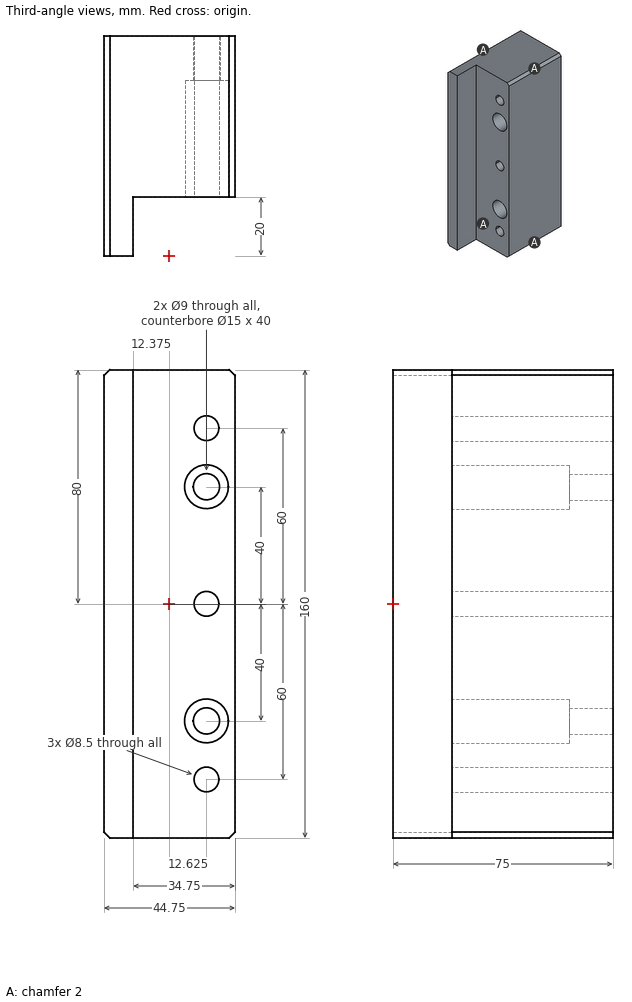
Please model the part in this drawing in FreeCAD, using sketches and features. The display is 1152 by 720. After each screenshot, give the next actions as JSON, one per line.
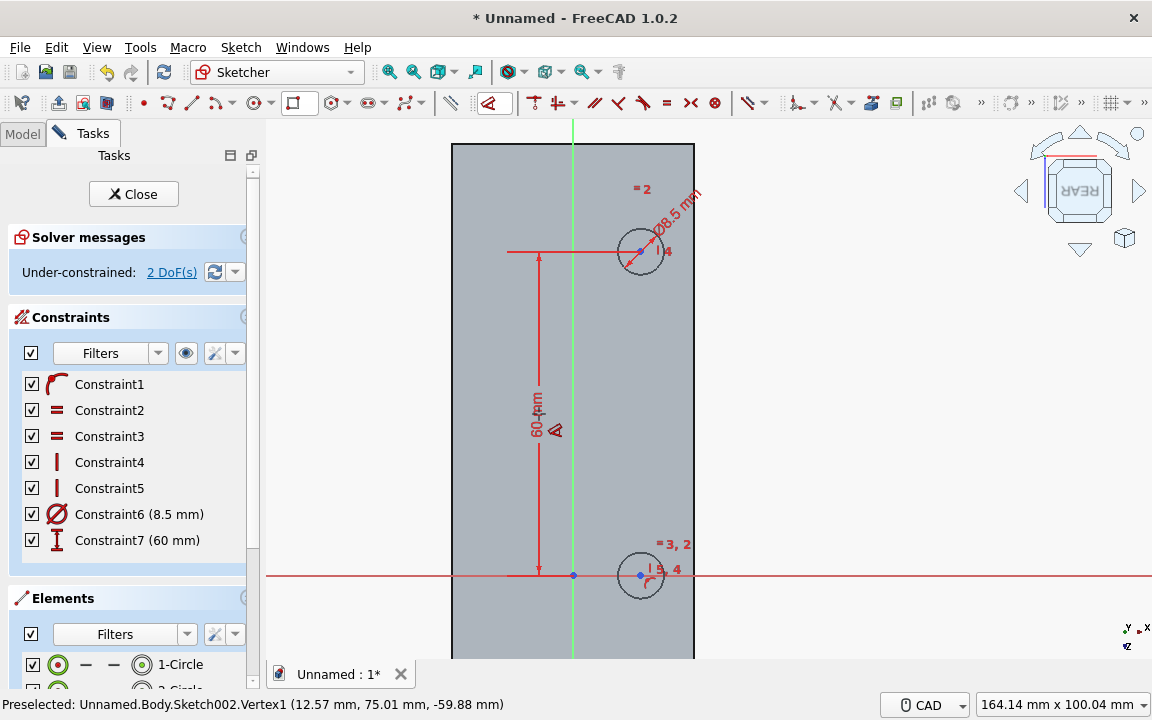
{"action": "scroll", "coordinate": [658, 237], "scroll_direction": "down", "scroll_amount": 4}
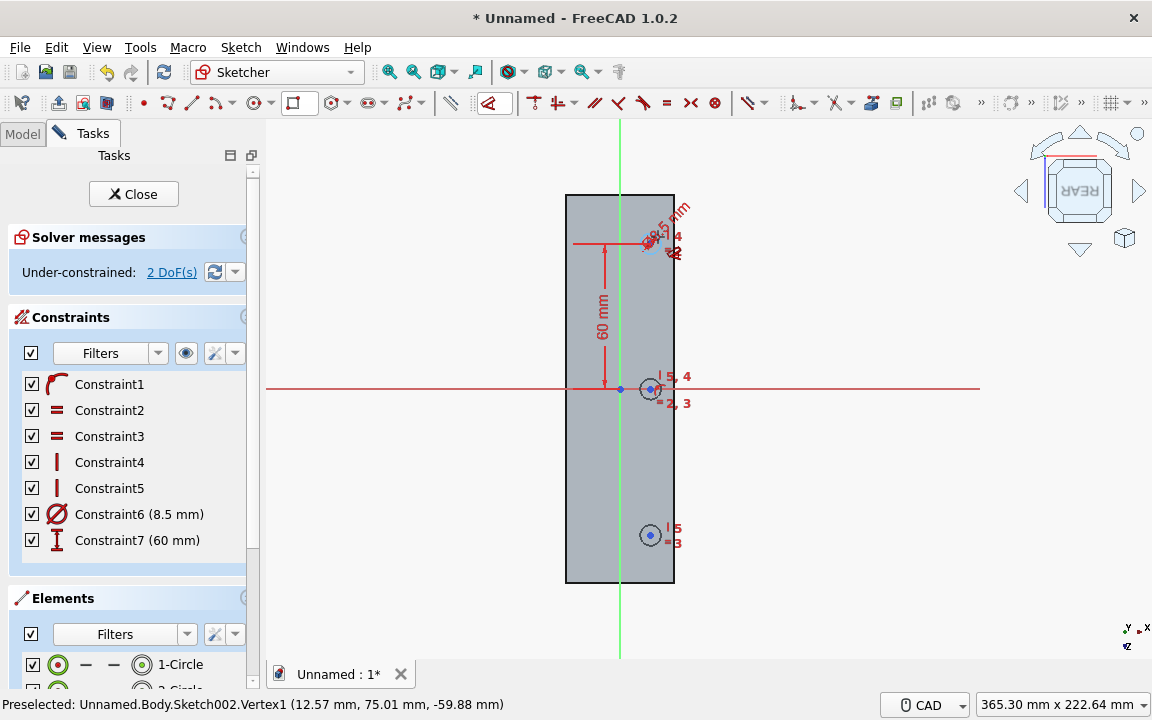
{"action": "left_click", "coordinate": [651, 535]}
{"action": "left_click", "coordinate": [586, 462]}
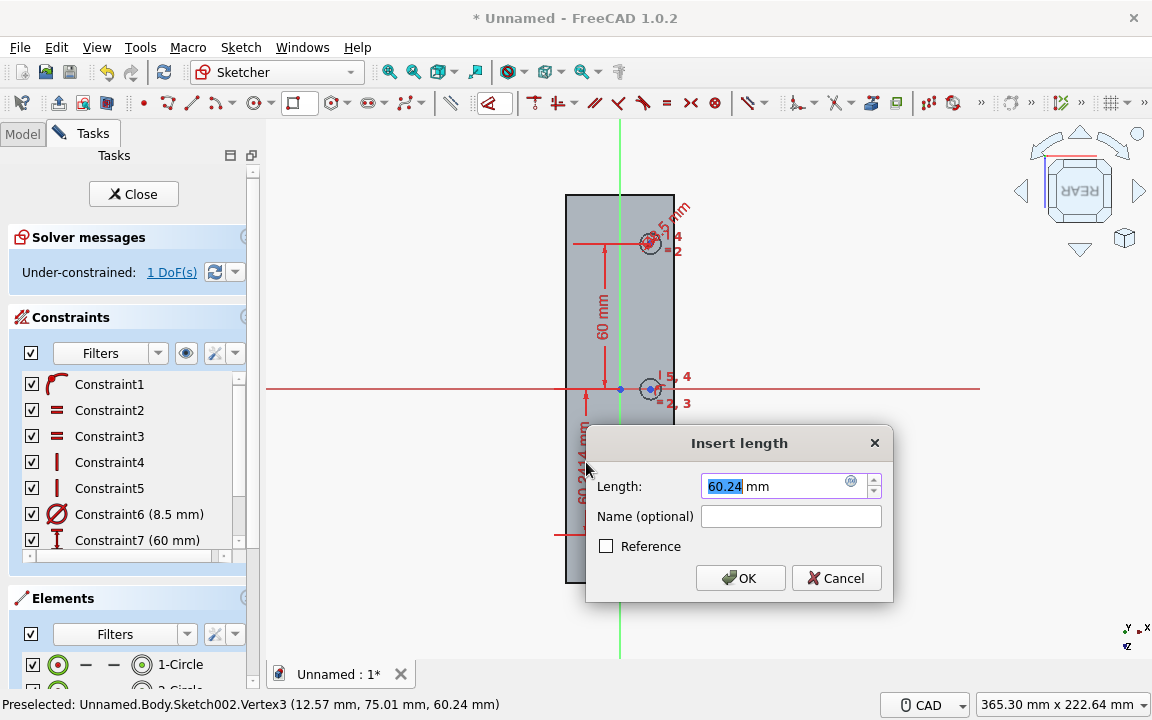
{"action": "type", "text": "60"}
{"action": "key", "text": "Return"}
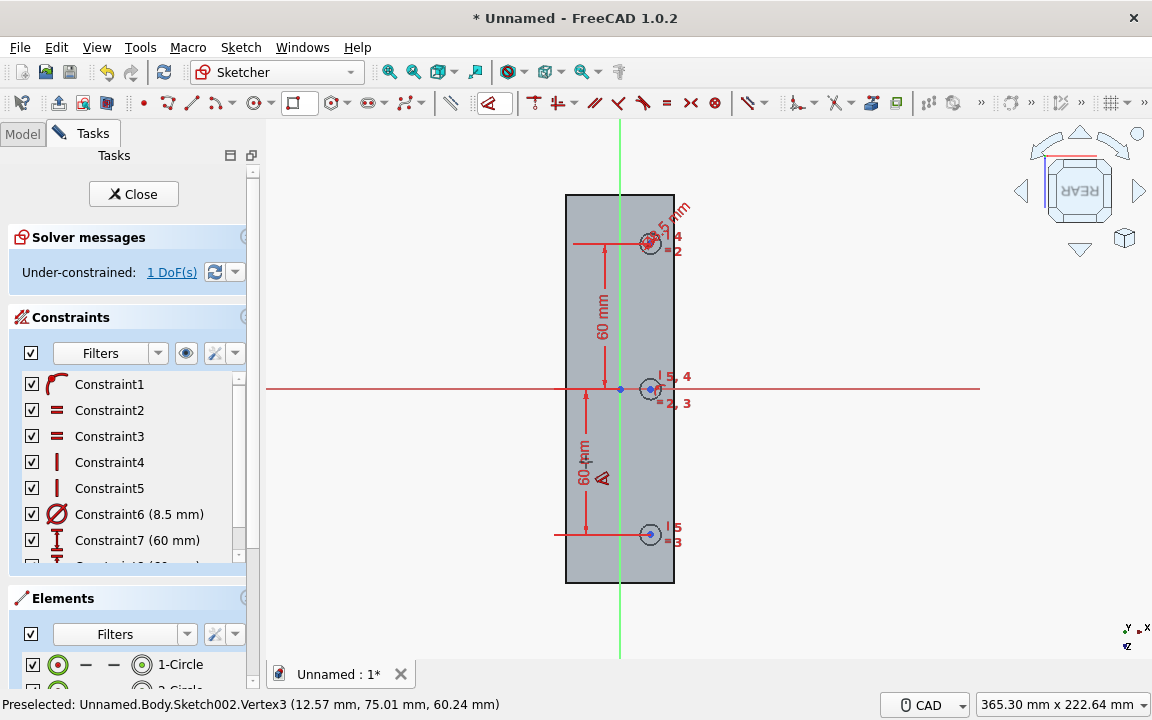
{"action": "scroll", "coordinate": [651, 244], "scroll_direction": "up", "scroll_amount": 2}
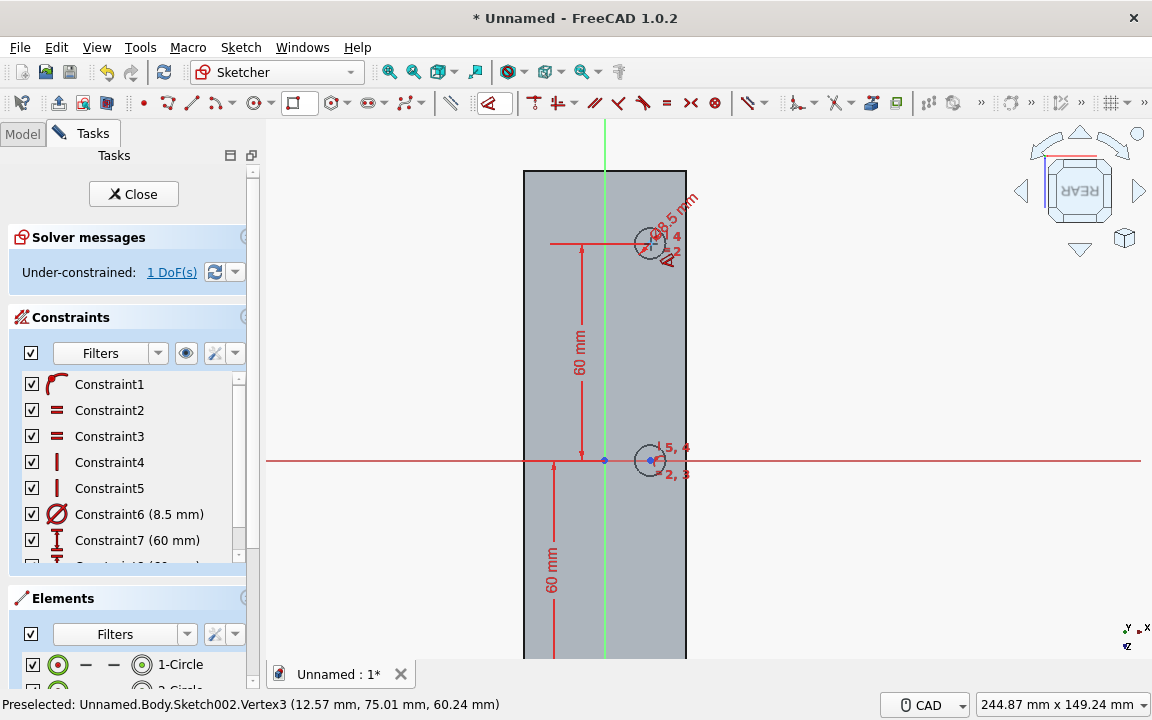
{"action": "left_click", "coordinate": [650, 244]}
{"action": "left_click", "coordinate": [627, 495]}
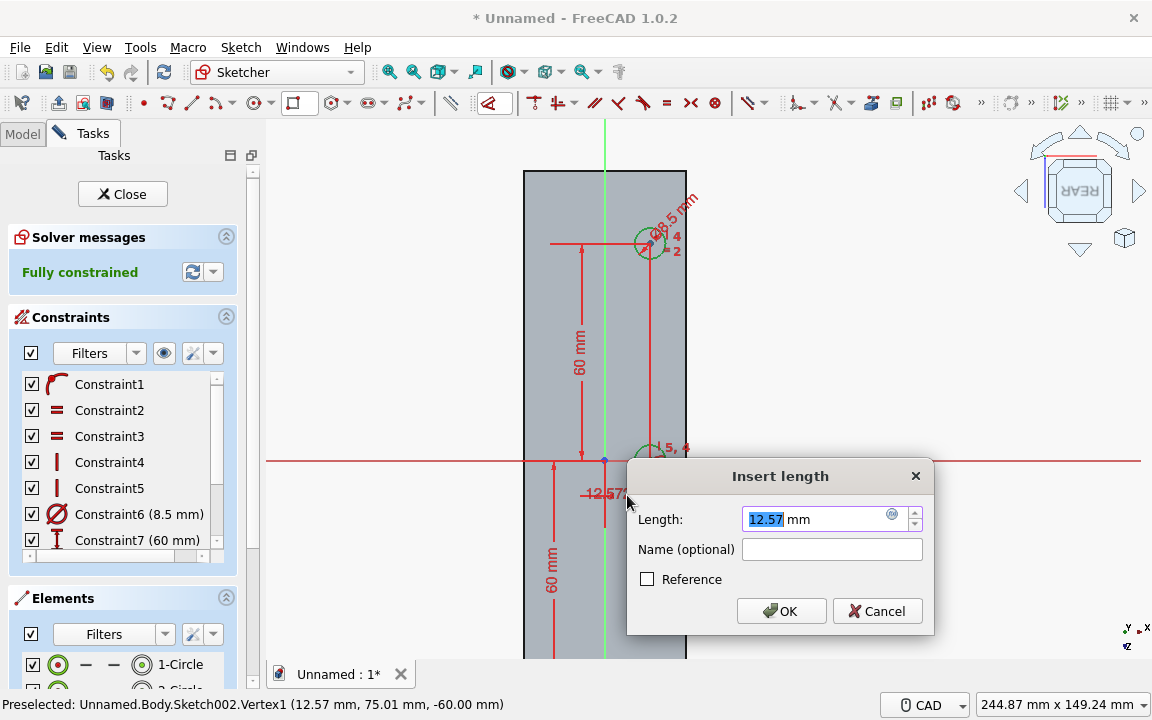
{"action": "type", "text": "12.625"}
{"action": "key", "text": "Return"}
{"action": "key", "text": "Escape"}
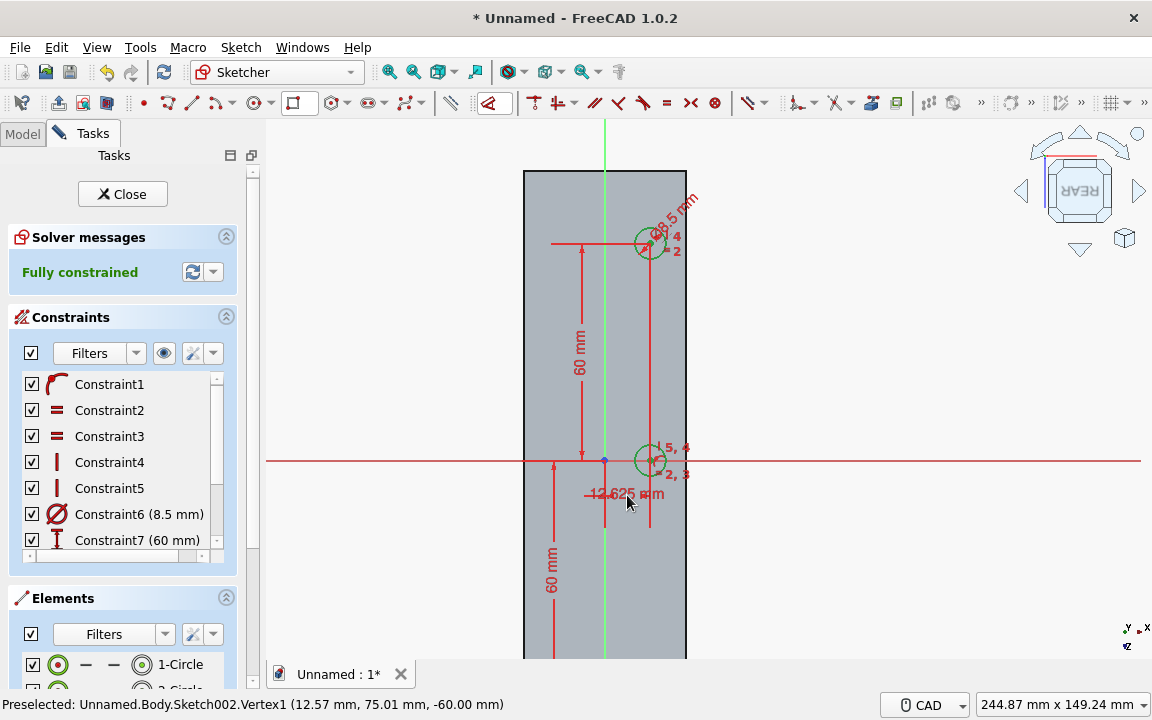
{"action": "left_click", "coordinate": [123, 194]}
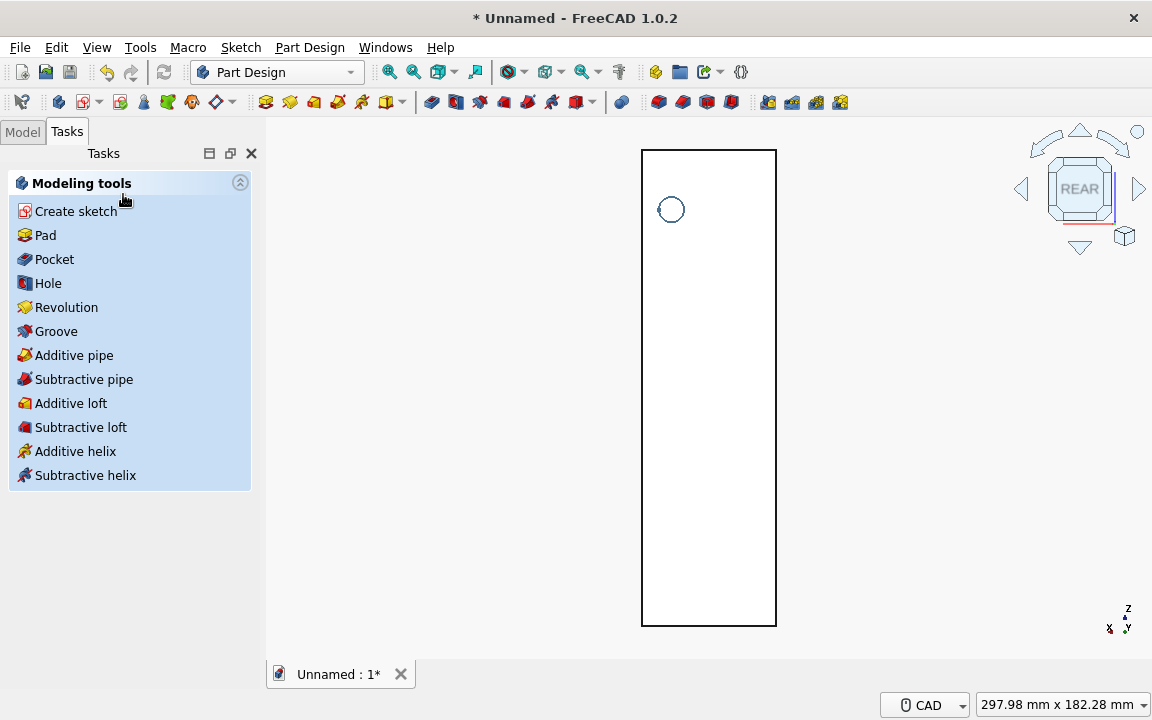
{"action": "left_click", "coordinate": [456, 102]}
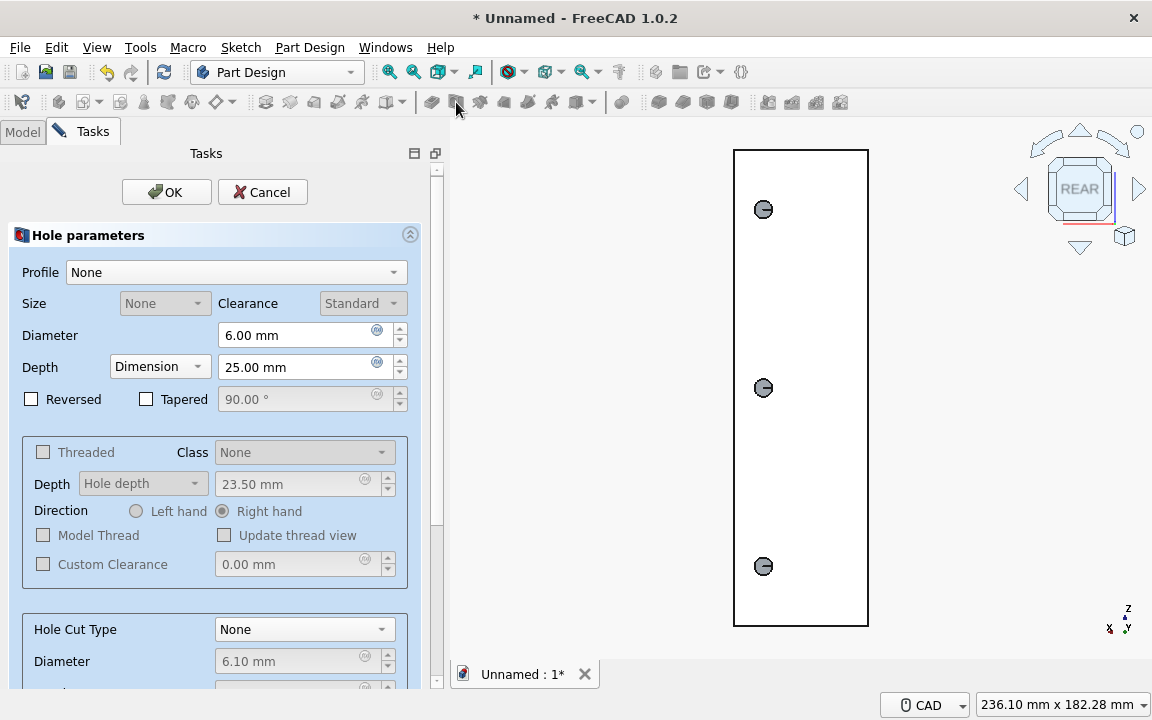
{"action": "triple_click", "coordinate": [305, 335]}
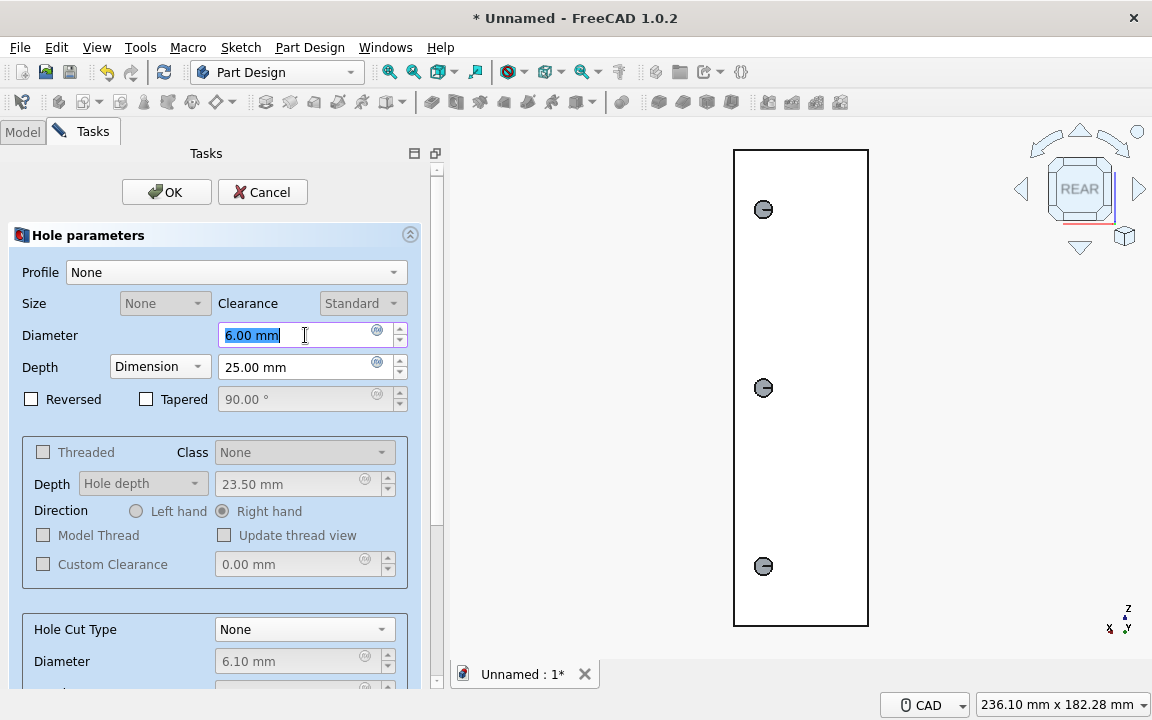
{"action": "type", "text": "8.5"}
{"action": "key", "text": "Tab"}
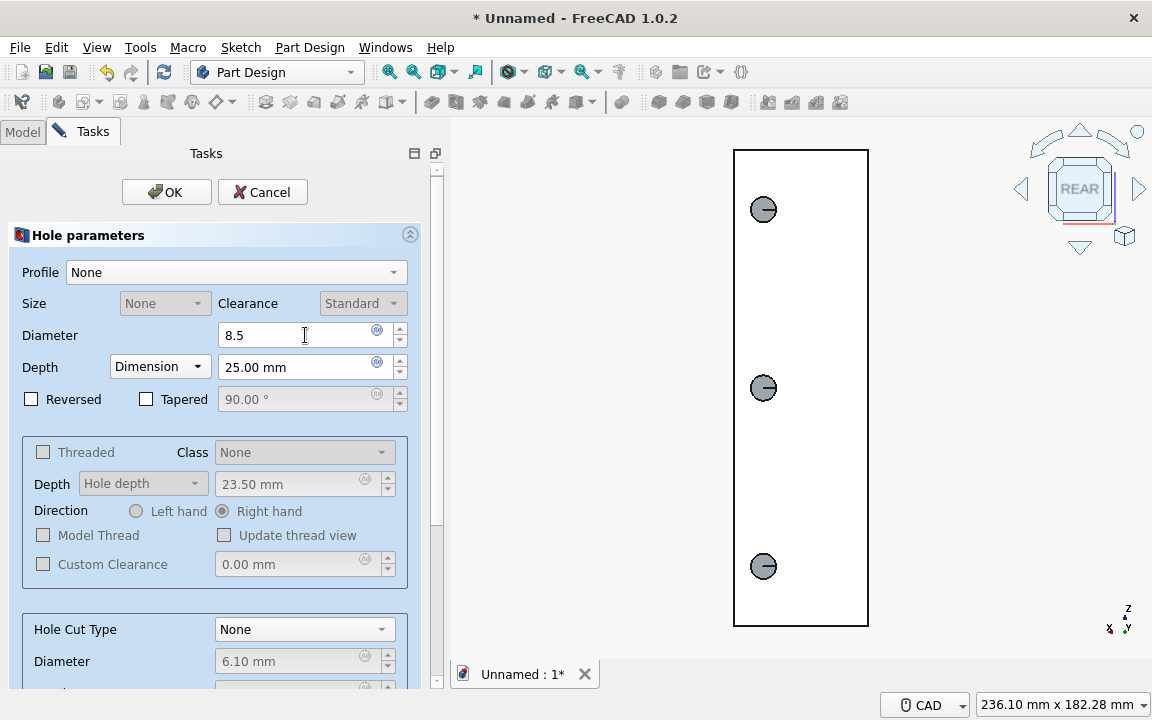
{"action": "left_click", "coordinate": [161, 366]}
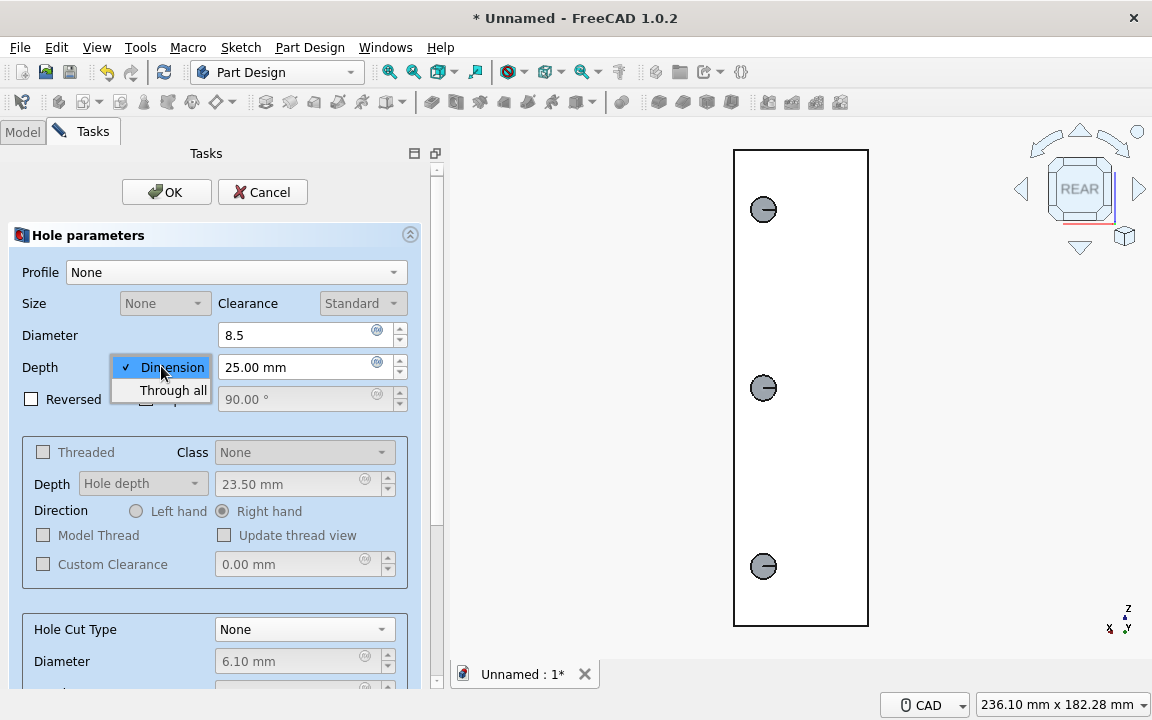
{"action": "left_click", "coordinate": [160, 390]}